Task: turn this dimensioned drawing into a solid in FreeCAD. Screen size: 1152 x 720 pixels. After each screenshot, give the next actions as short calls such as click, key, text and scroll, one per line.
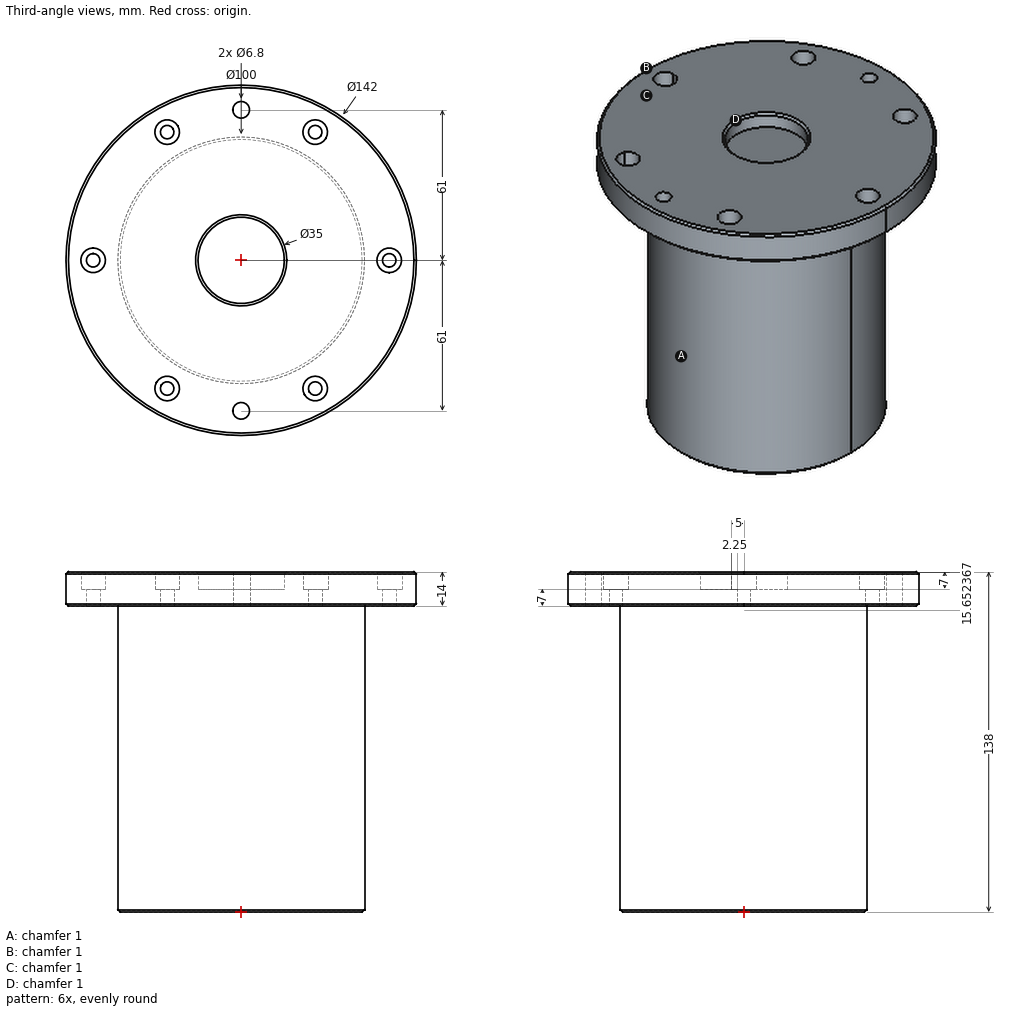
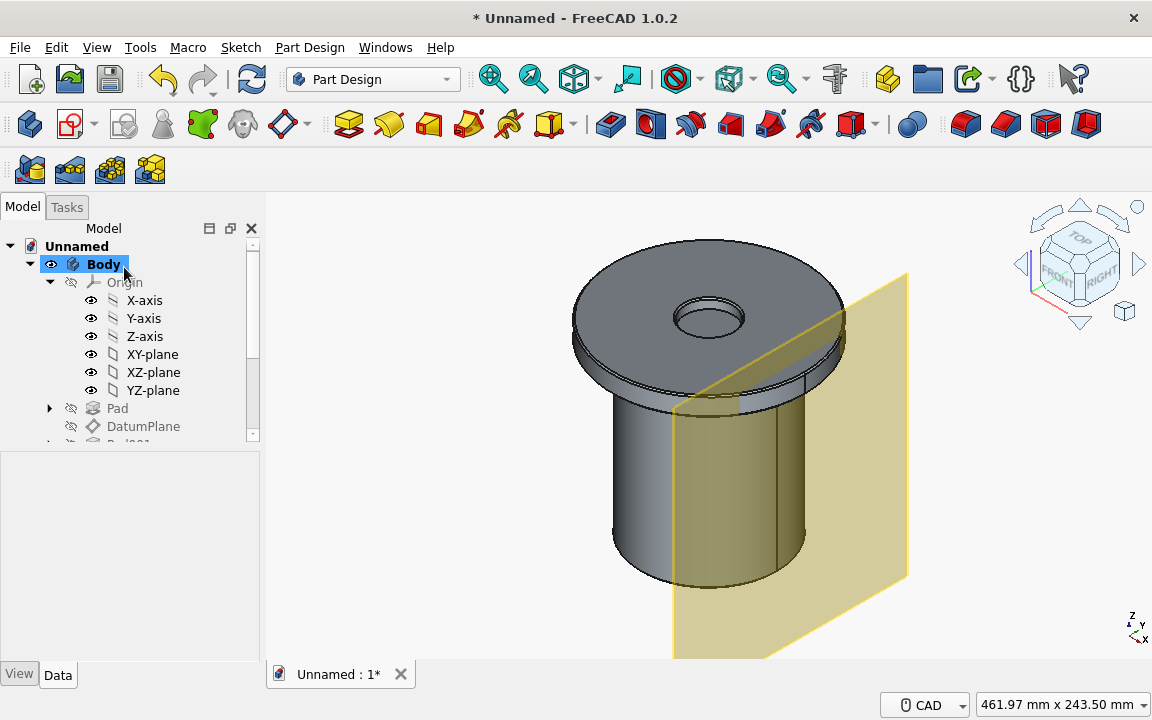
scroll(100, 332, down, 3)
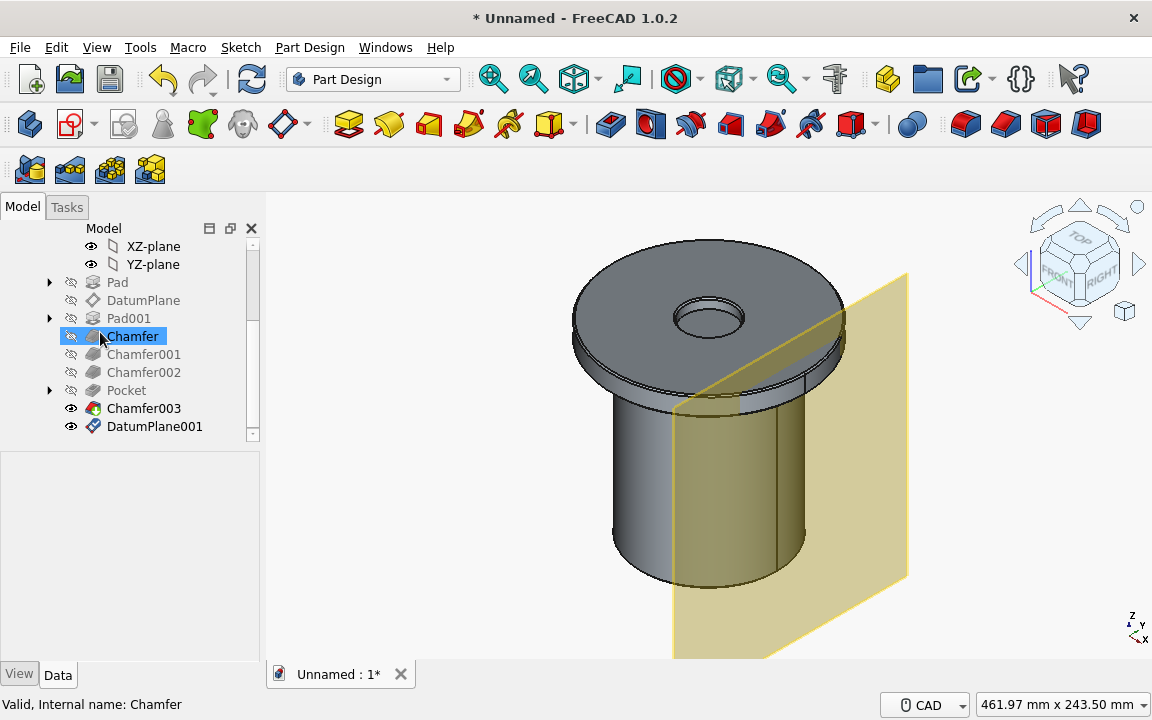
click(116, 426)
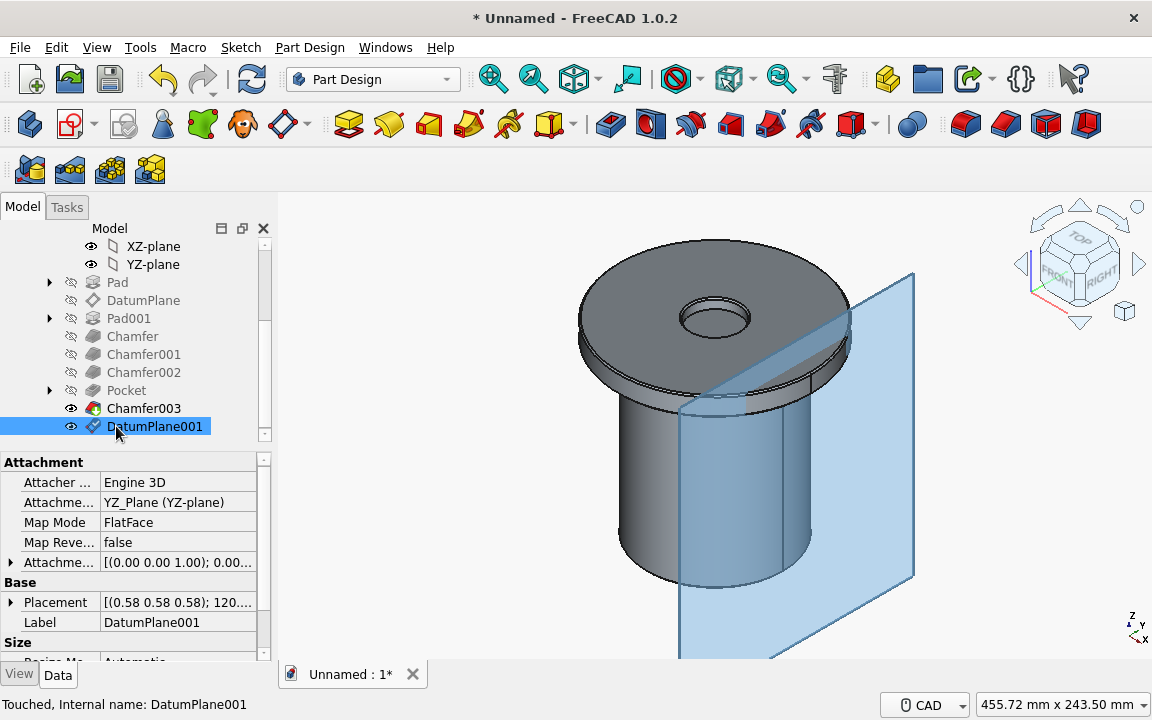
click(70, 124)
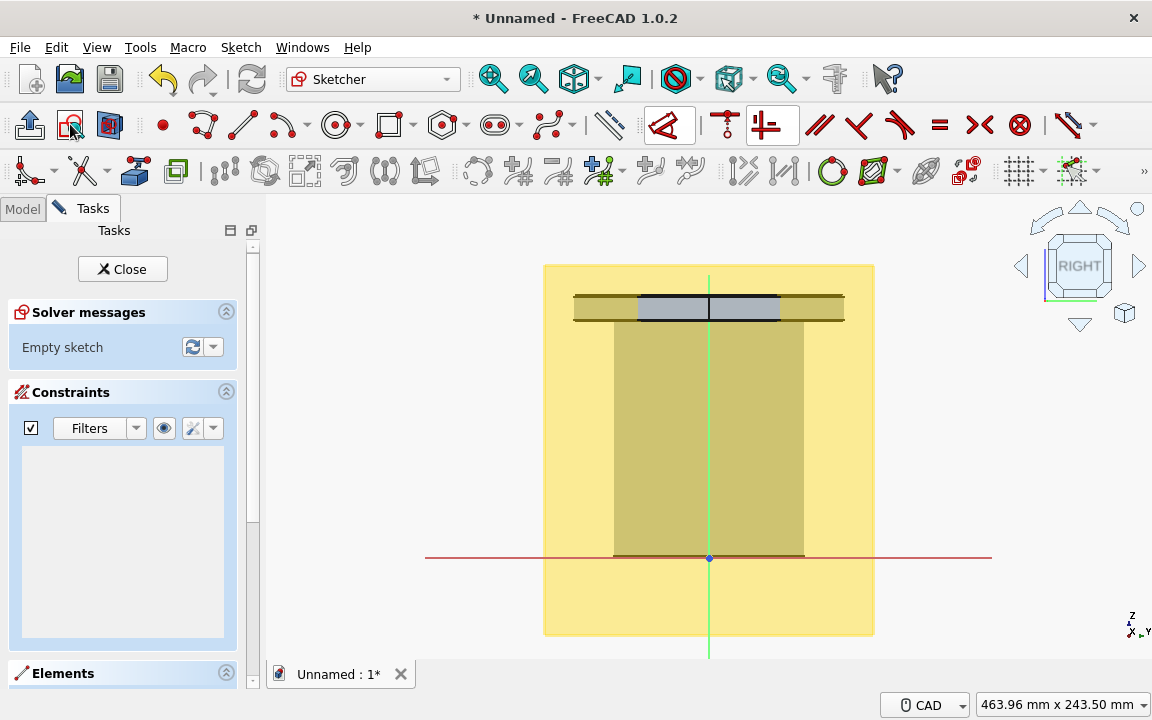
click(110, 126)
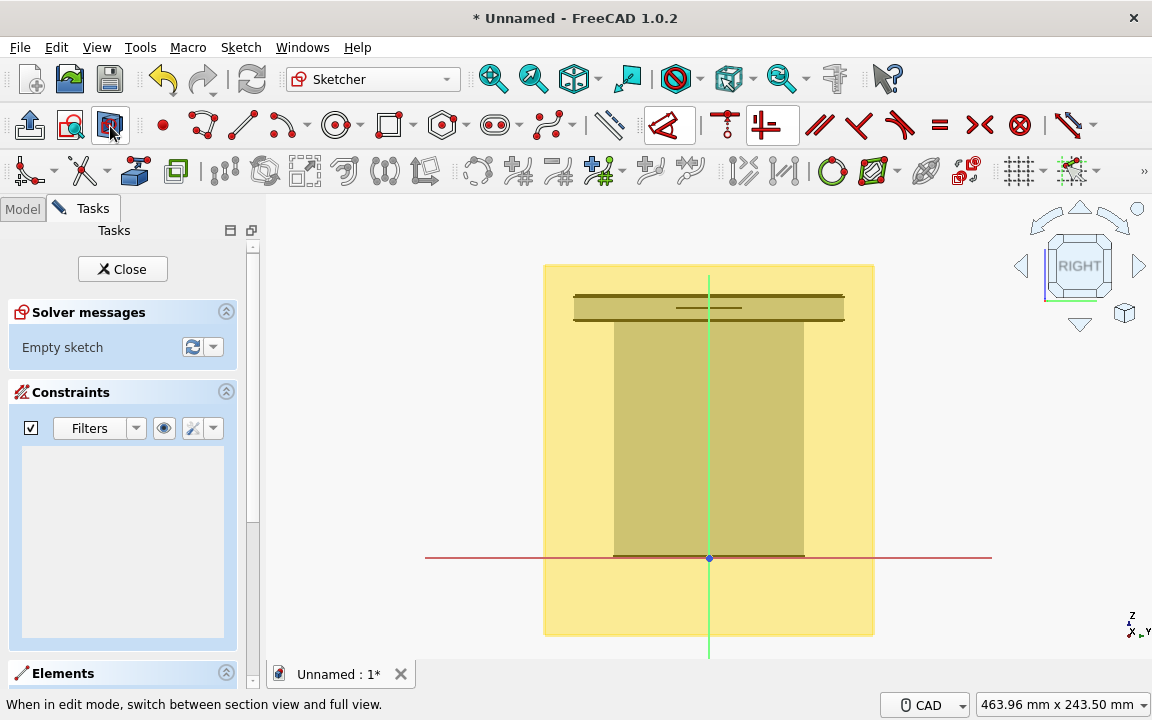
scroll(712, 295, up, 11)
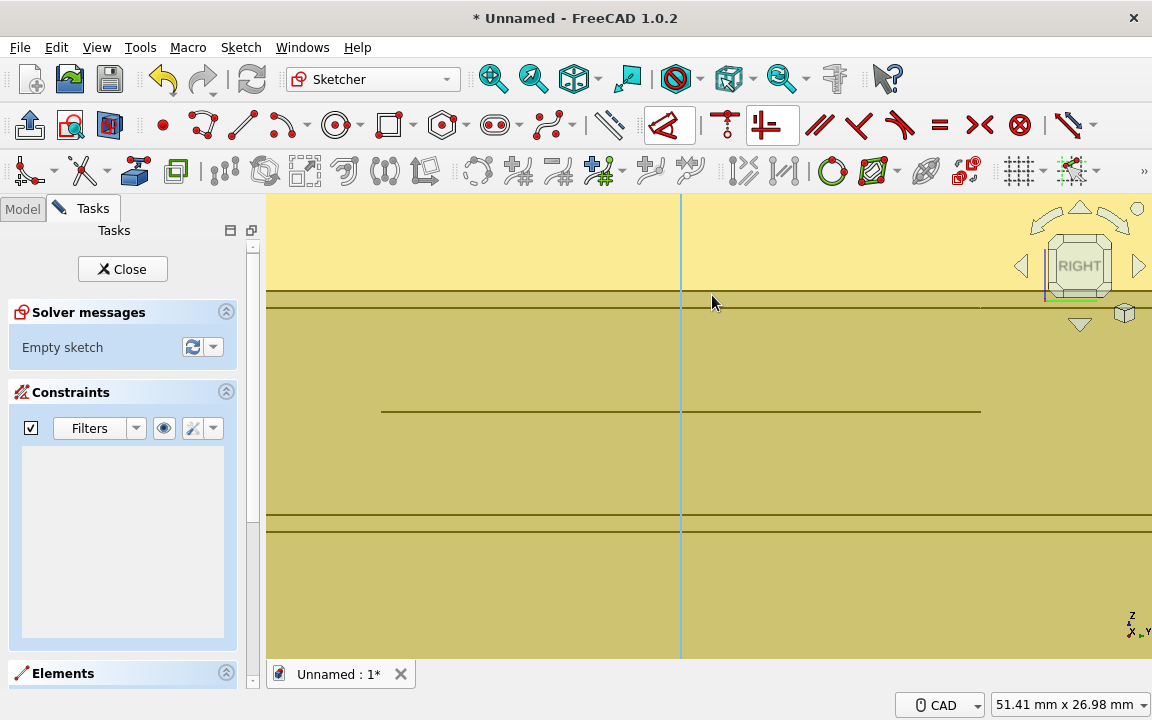
key(g)
key(m)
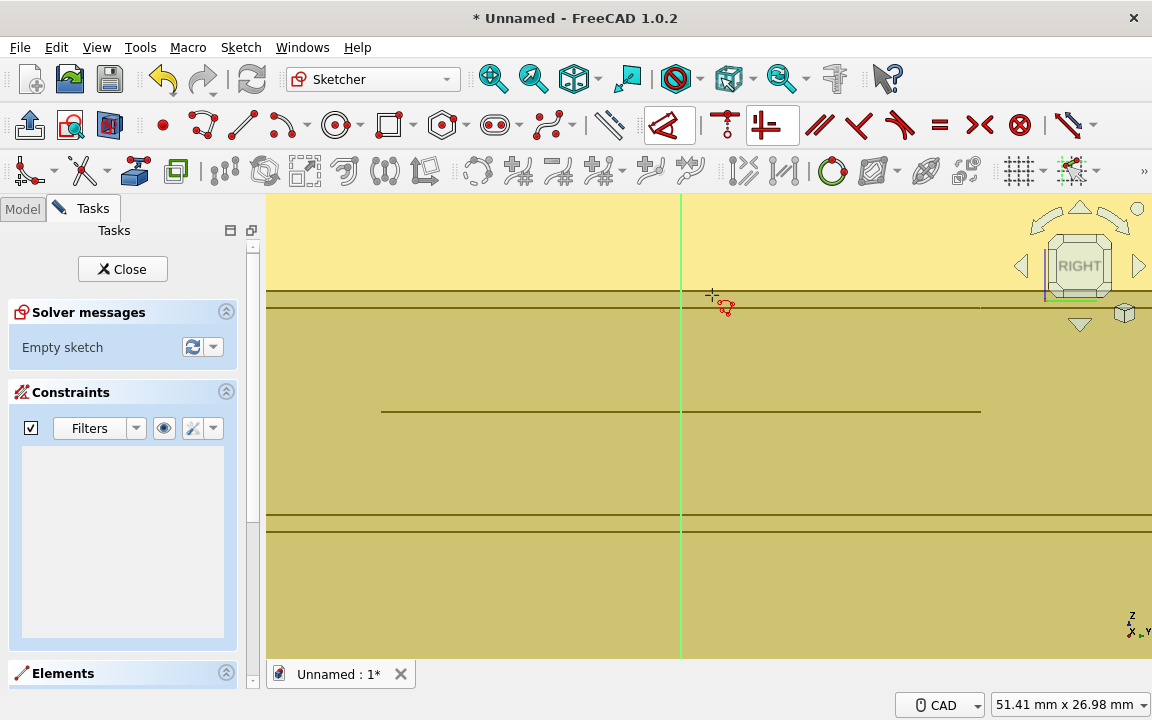
click(681, 561)
click(672, 291)
click(595, 291)
click(595, 411)
click(633, 411)
click(633, 532)
click(681, 562)
key(Escape)
key(Escape)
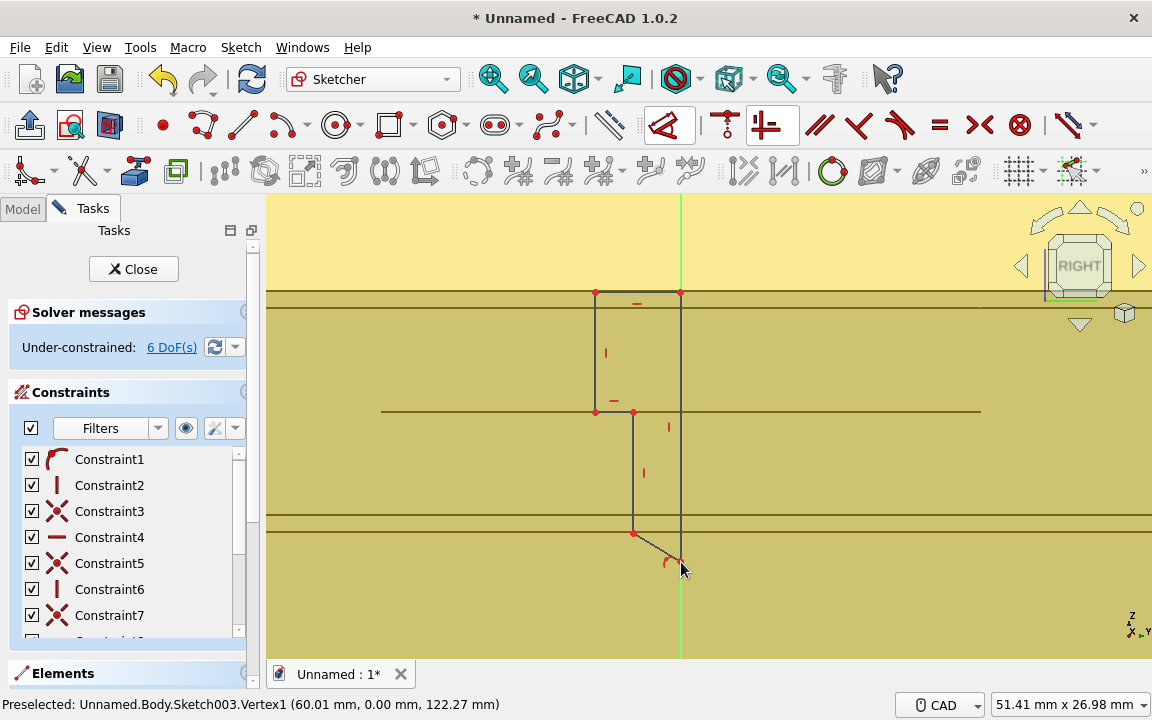
click(655, 292)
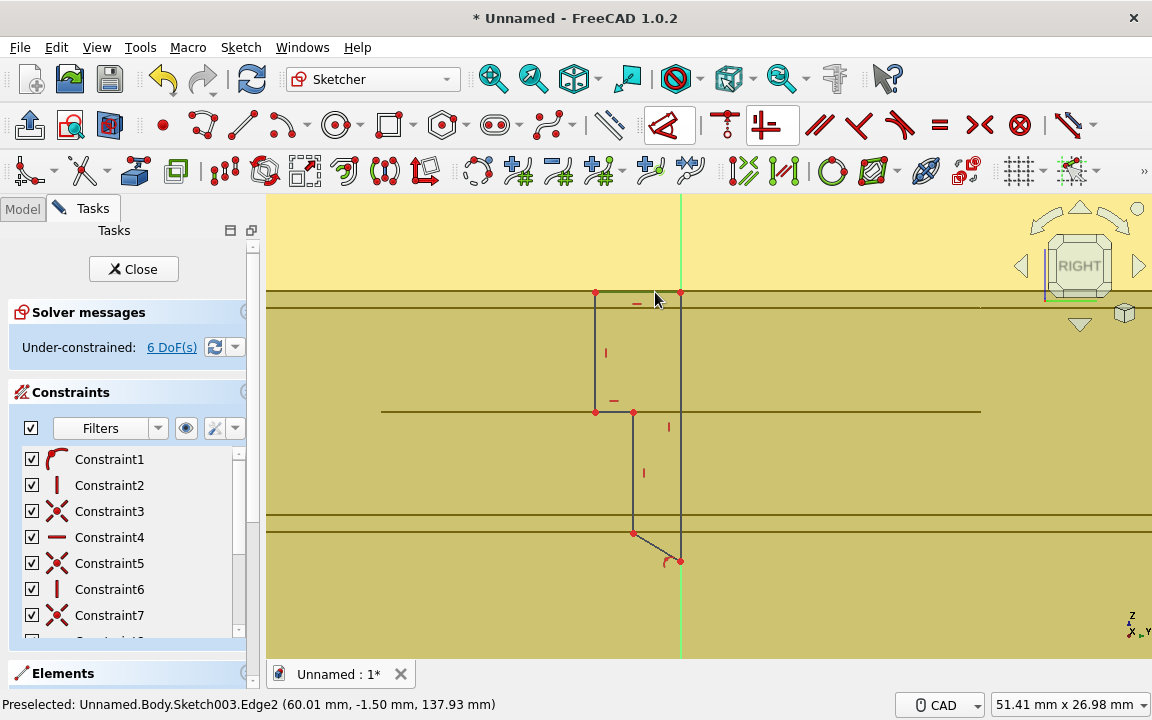
key(l)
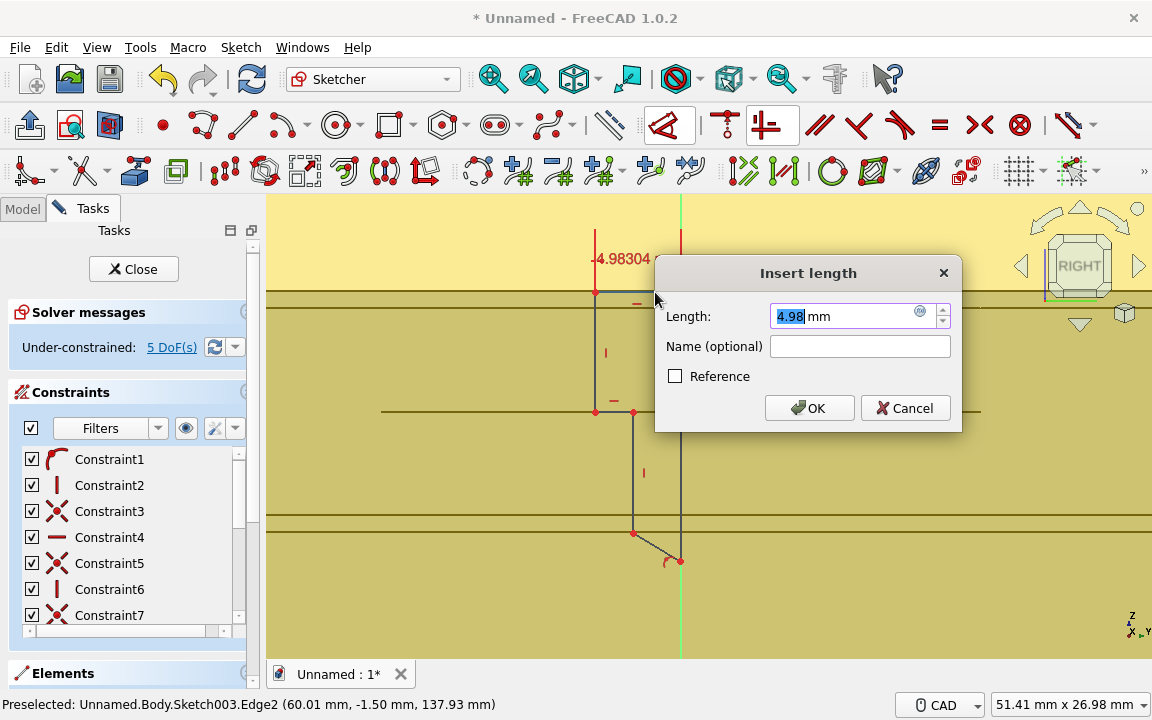
text(5)
key(Return)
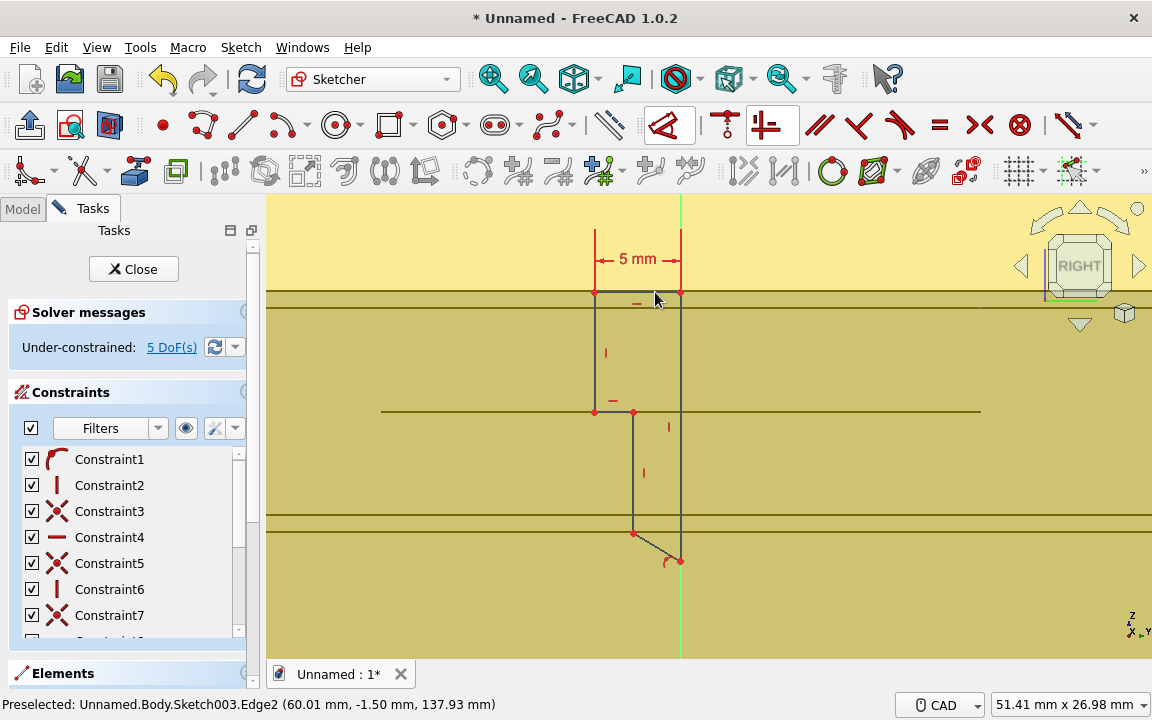
click(595, 328)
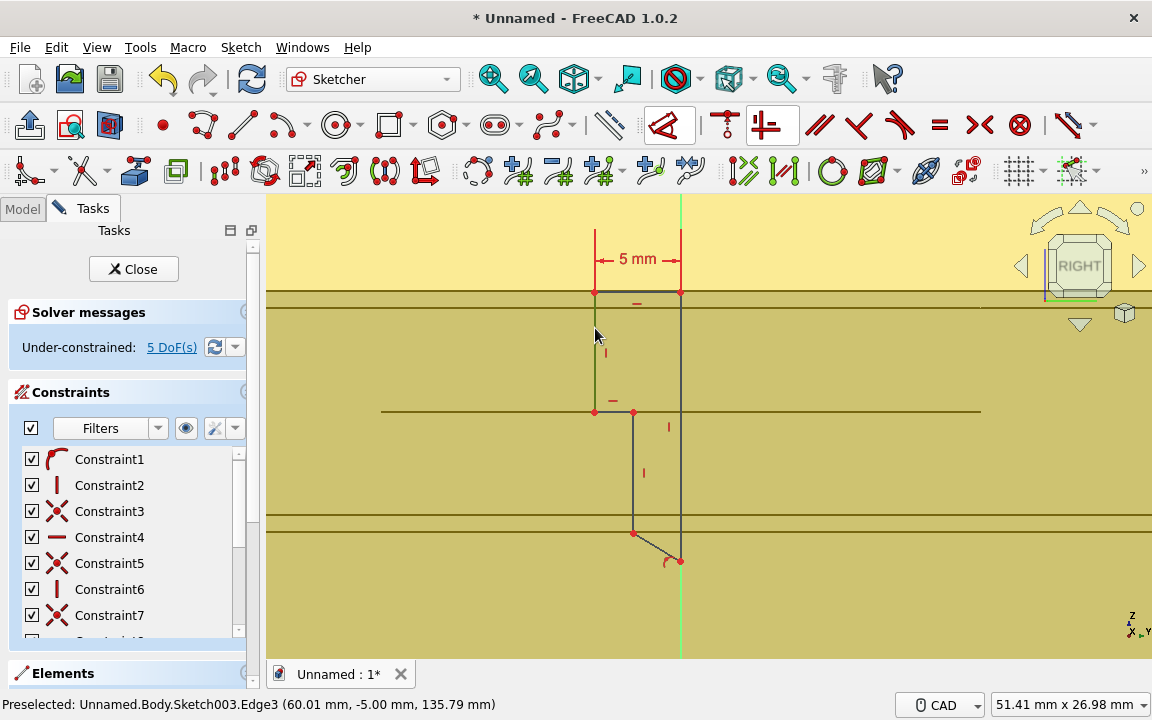
key(i)